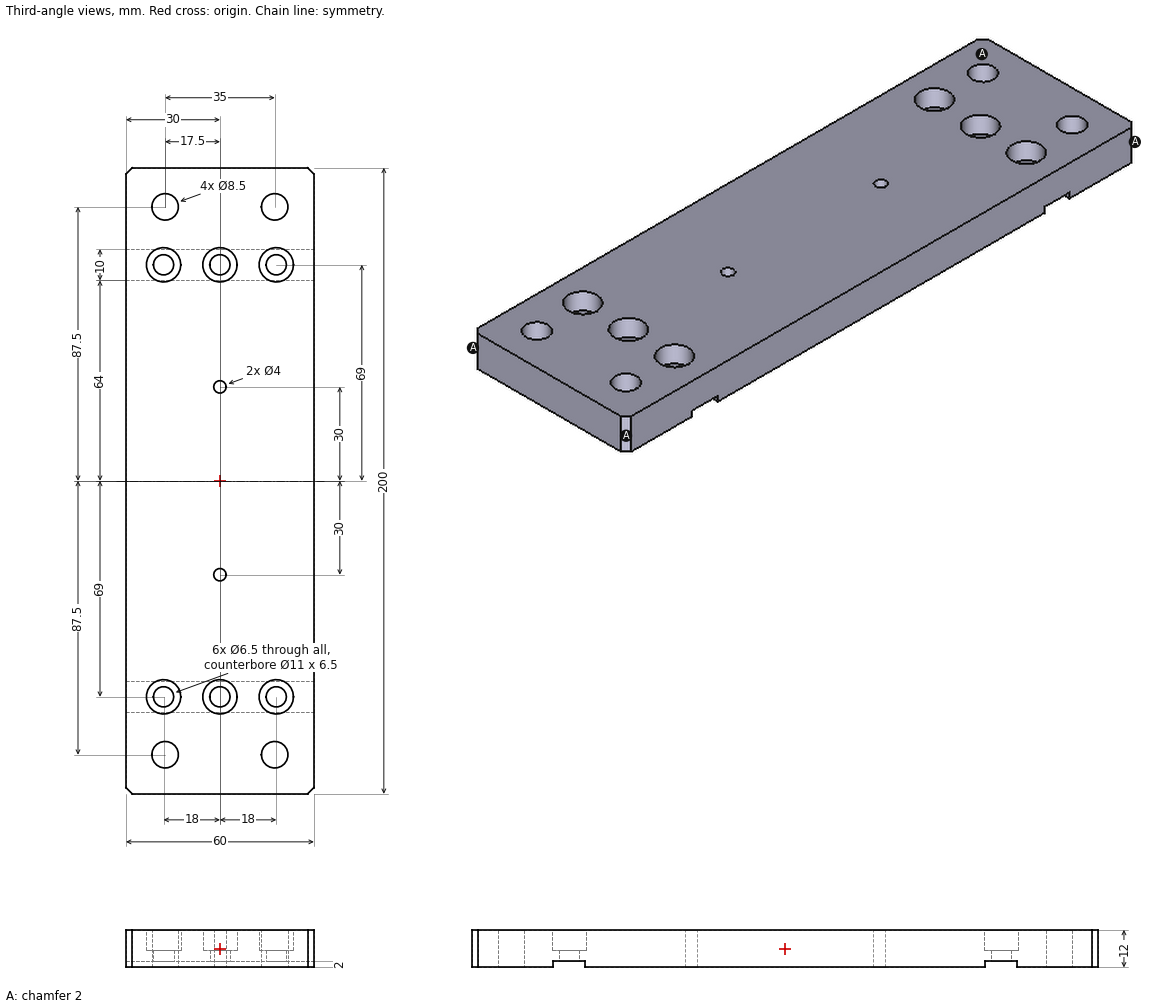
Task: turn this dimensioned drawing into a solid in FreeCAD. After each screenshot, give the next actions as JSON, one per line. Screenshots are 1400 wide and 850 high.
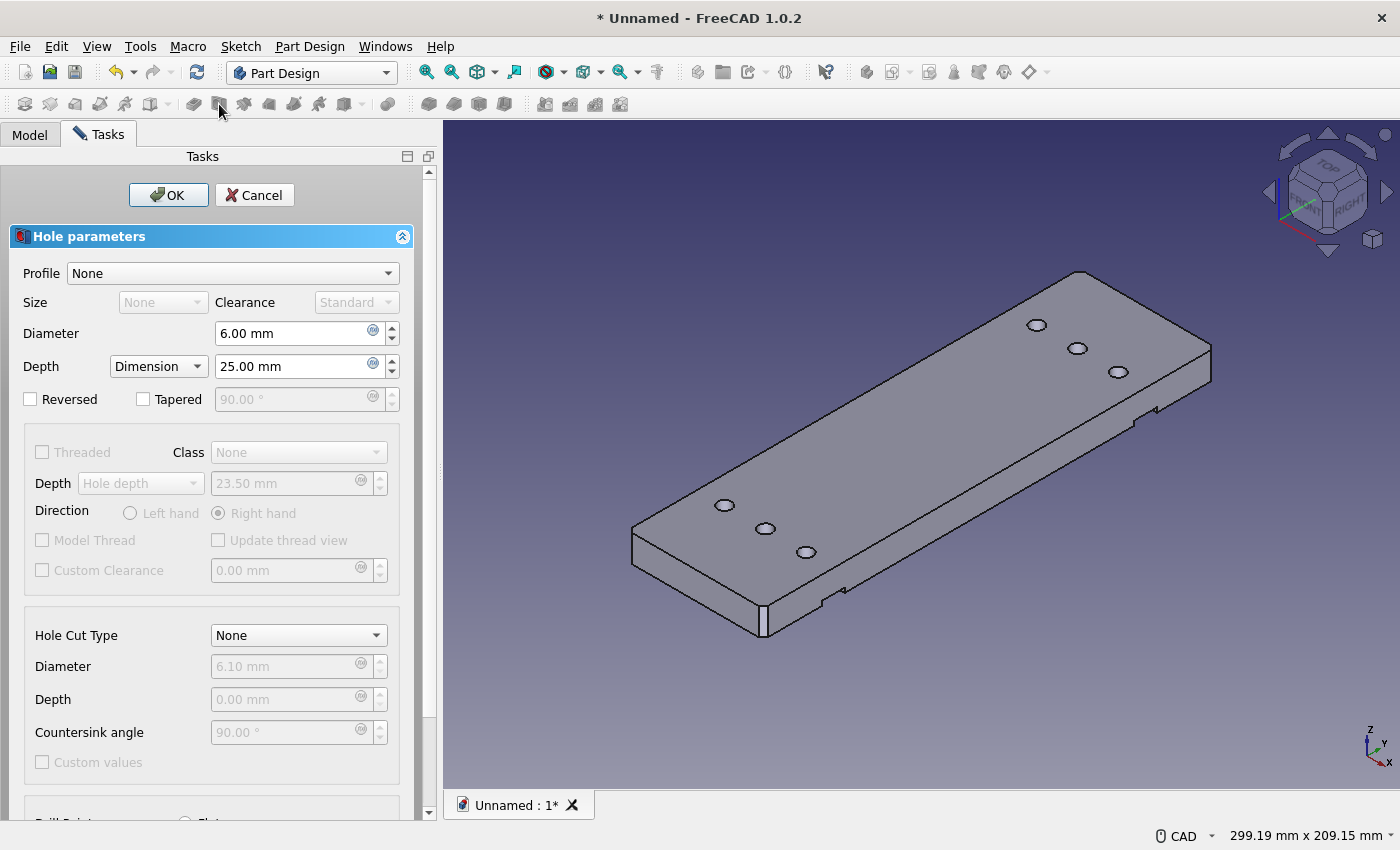
{"action": "triple_click", "coordinate": [300, 334]}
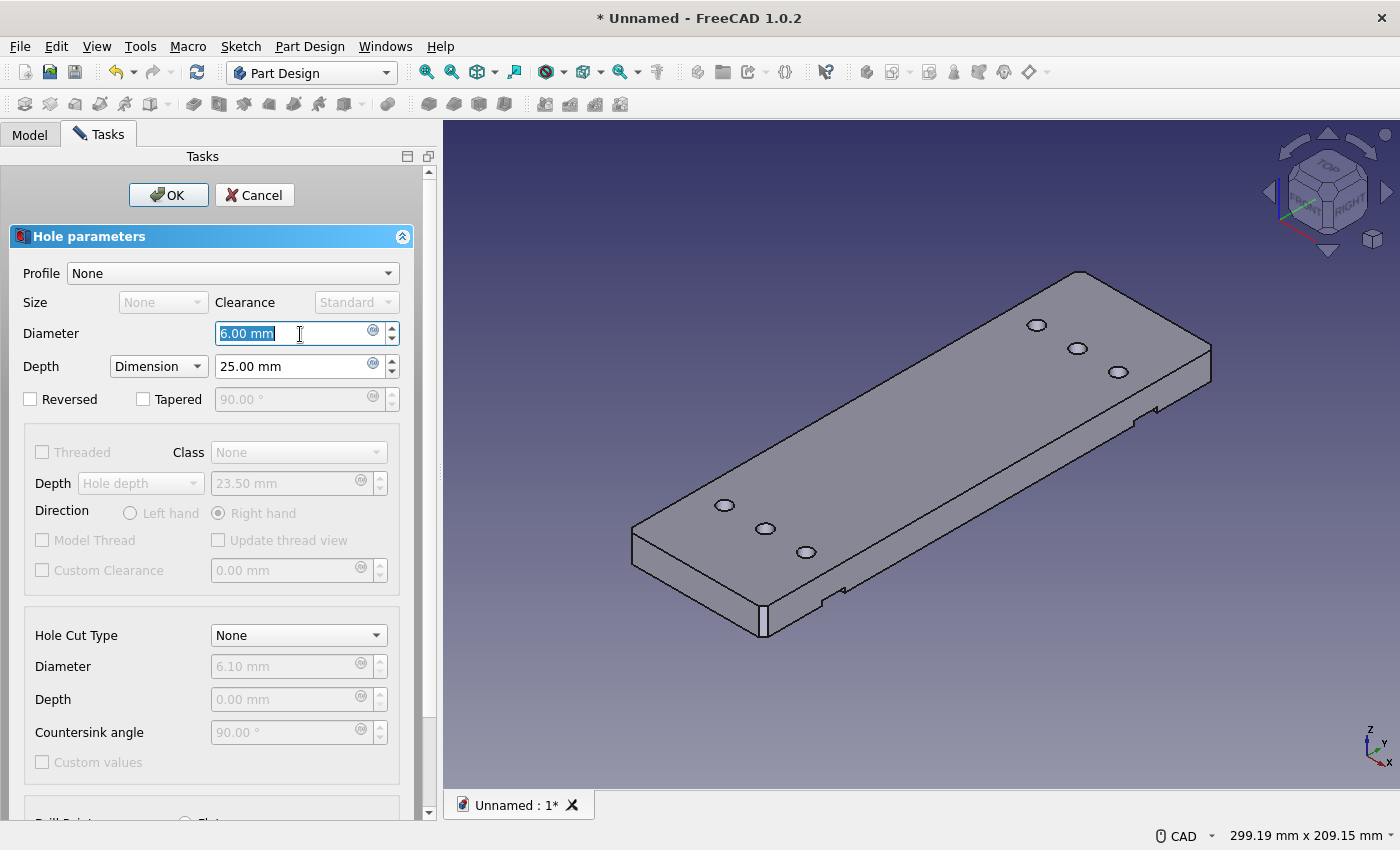
{"action": "type", "text": "6.5"}
{"action": "key", "text": "Tab"}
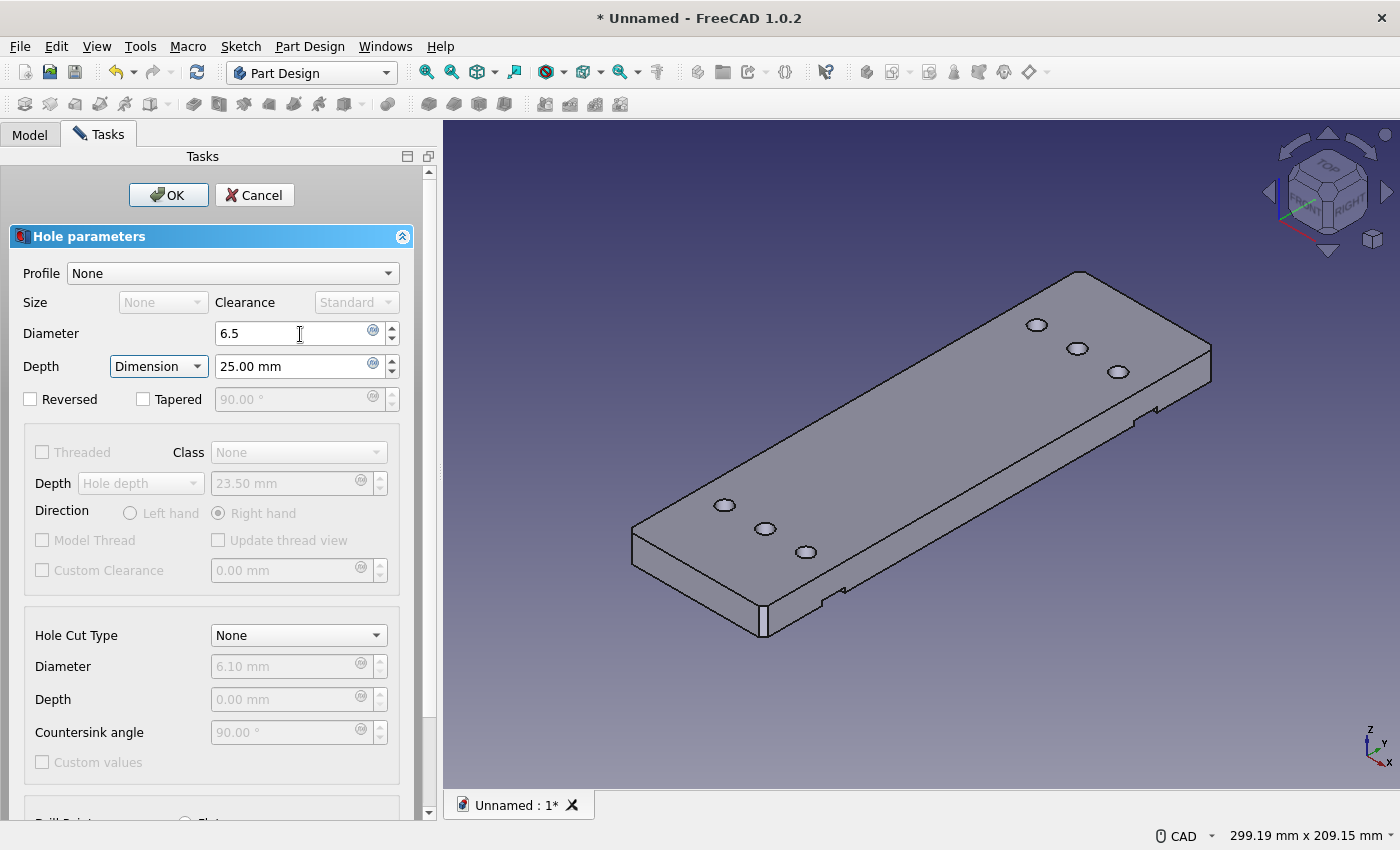
{"action": "left_click", "coordinate": [160, 366]}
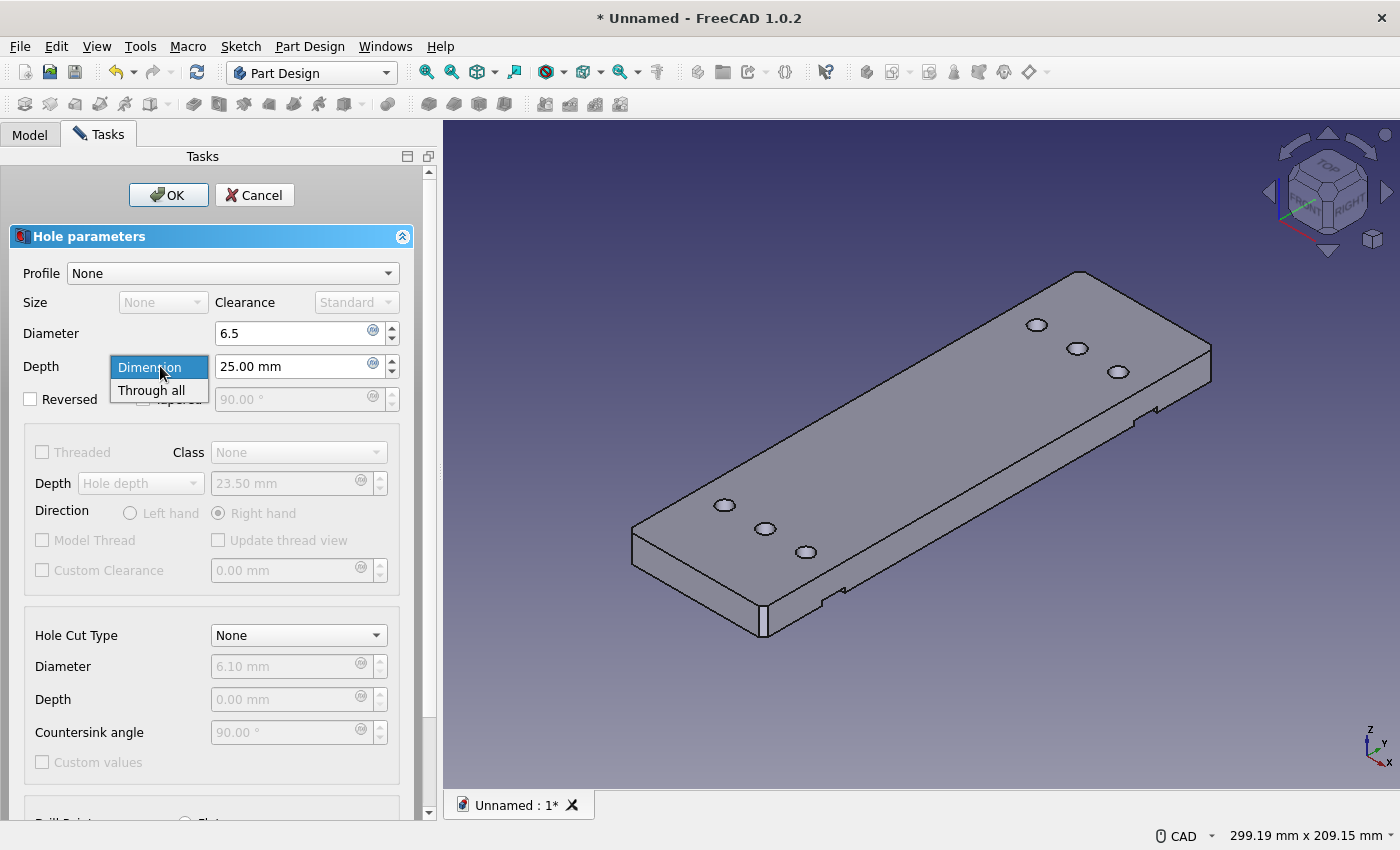
{"action": "left_click", "coordinate": [158, 390]}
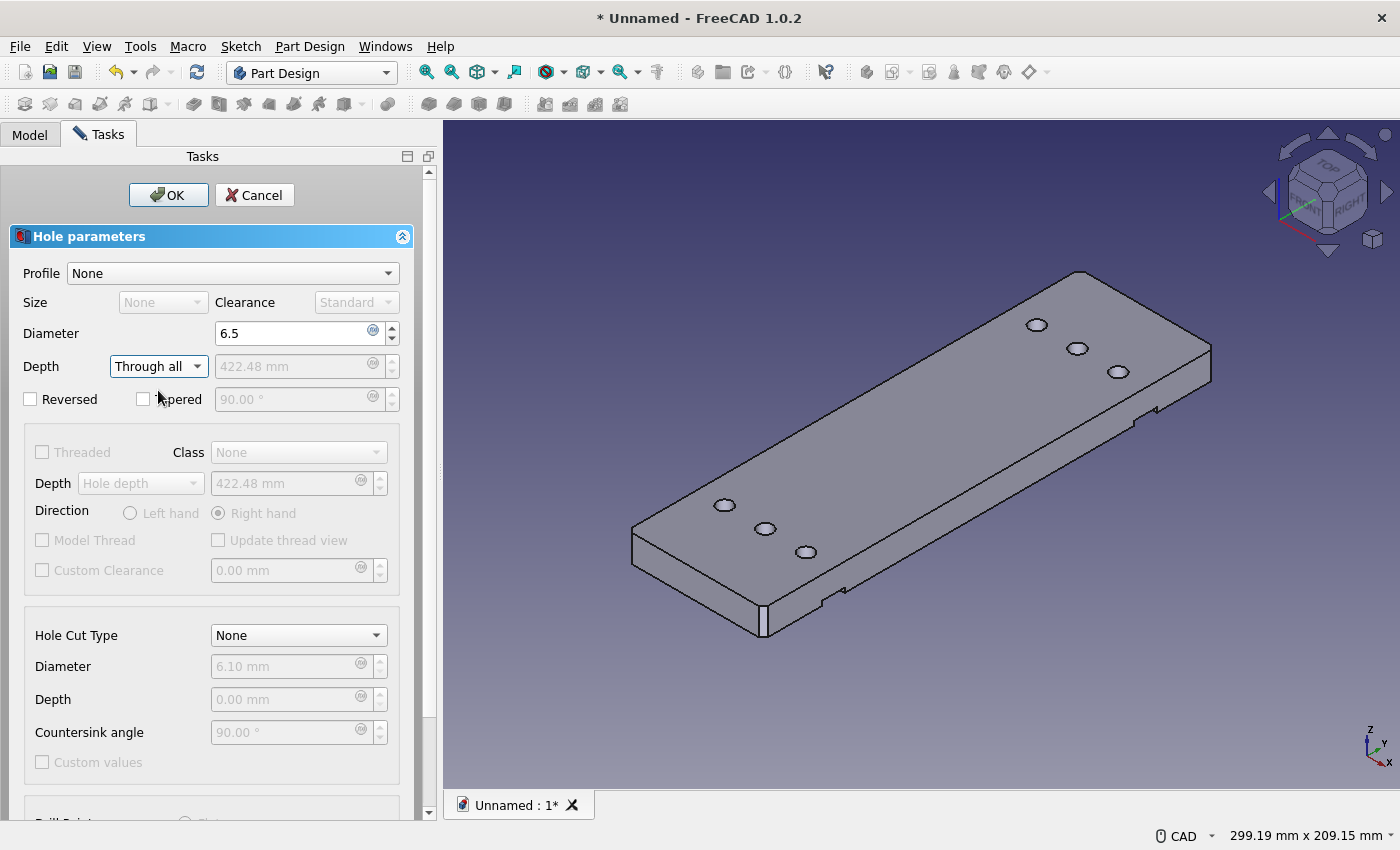
{"action": "left_click", "coordinate": [300, 636]}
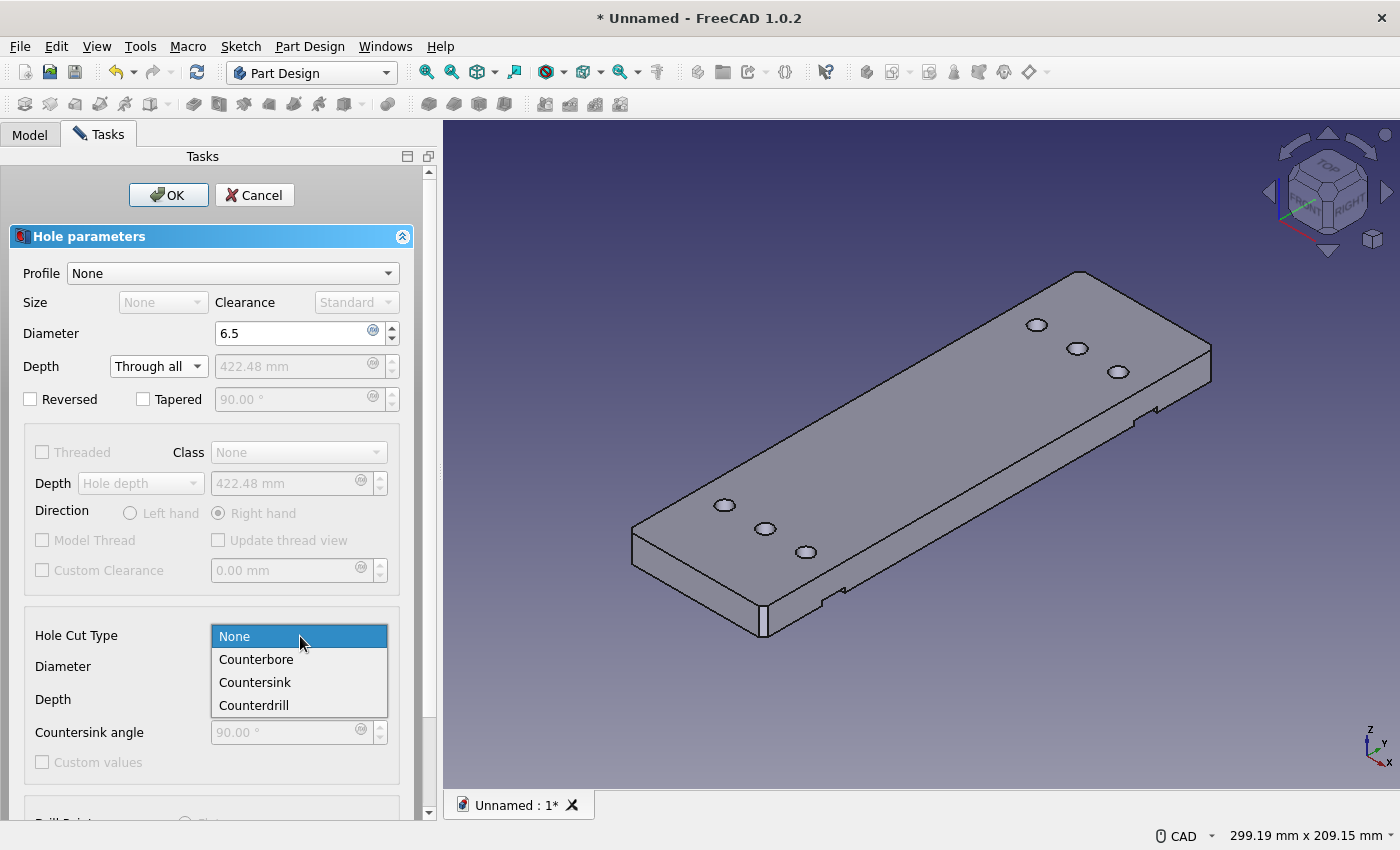
{"action": "left_click", "coordinate": [298, 660]}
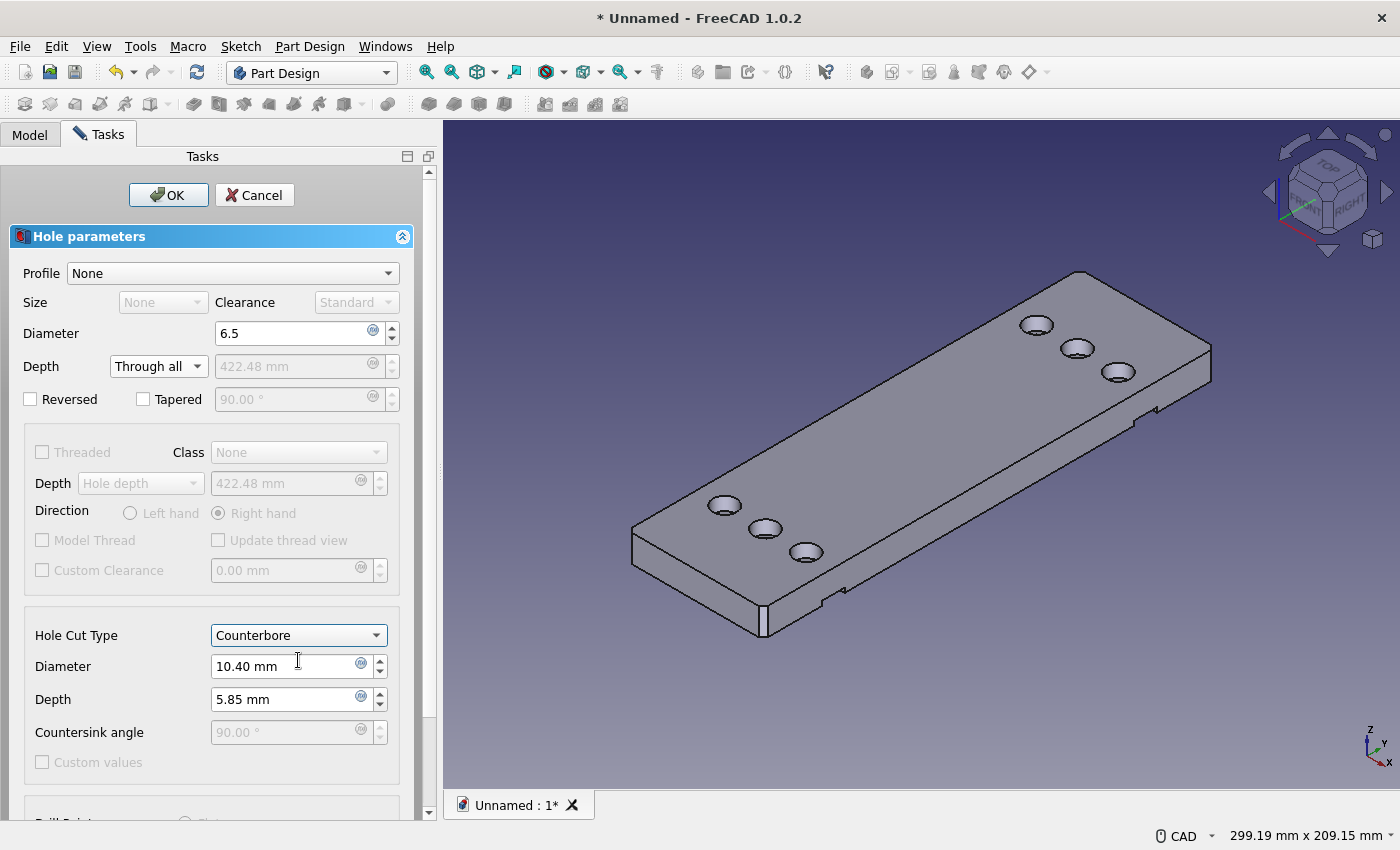
{"action": "triple_click", "coordinate": [292, 666]}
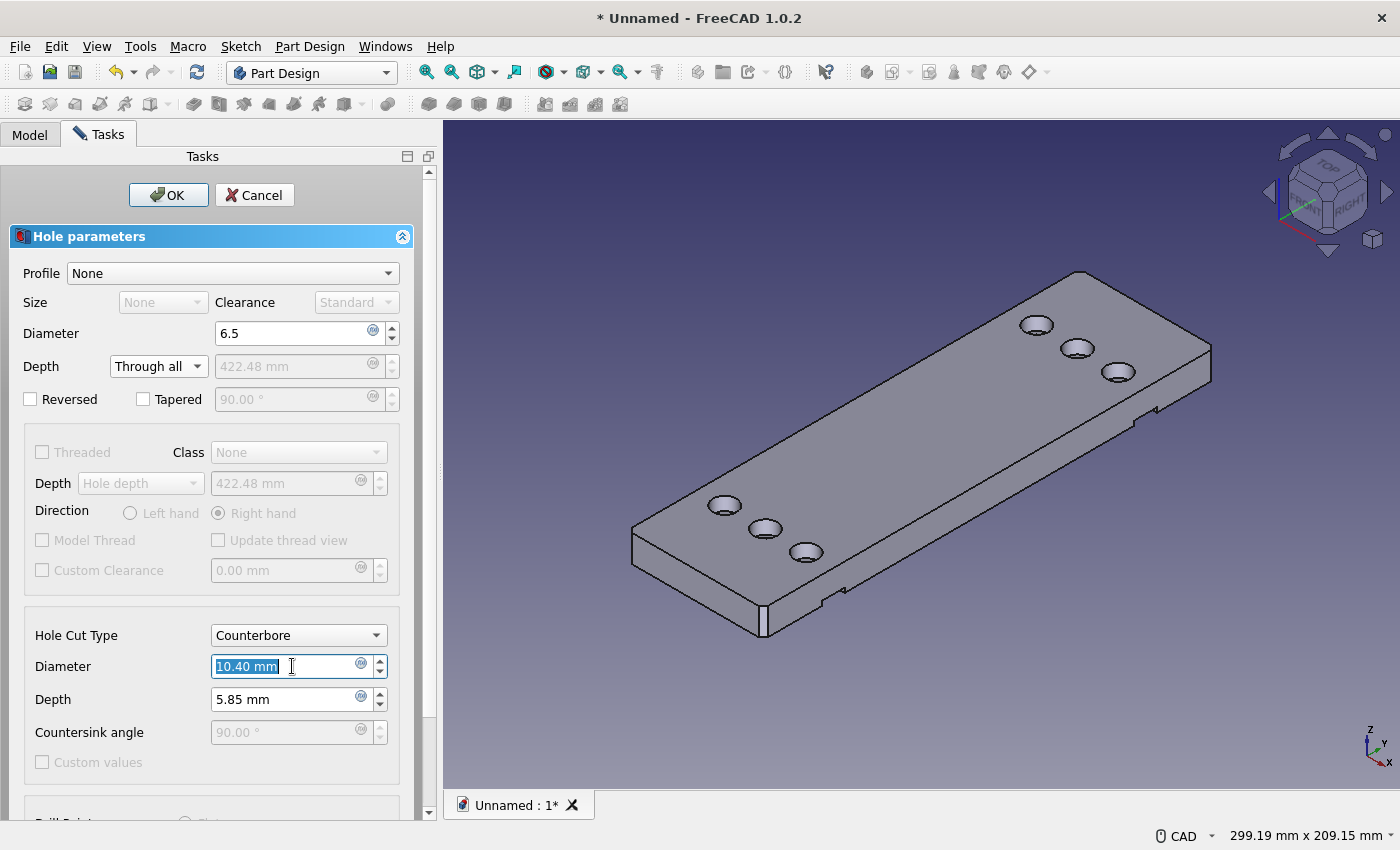
{"action": "type", "text": "11"}
{"action": "key", "text": "Tab"}